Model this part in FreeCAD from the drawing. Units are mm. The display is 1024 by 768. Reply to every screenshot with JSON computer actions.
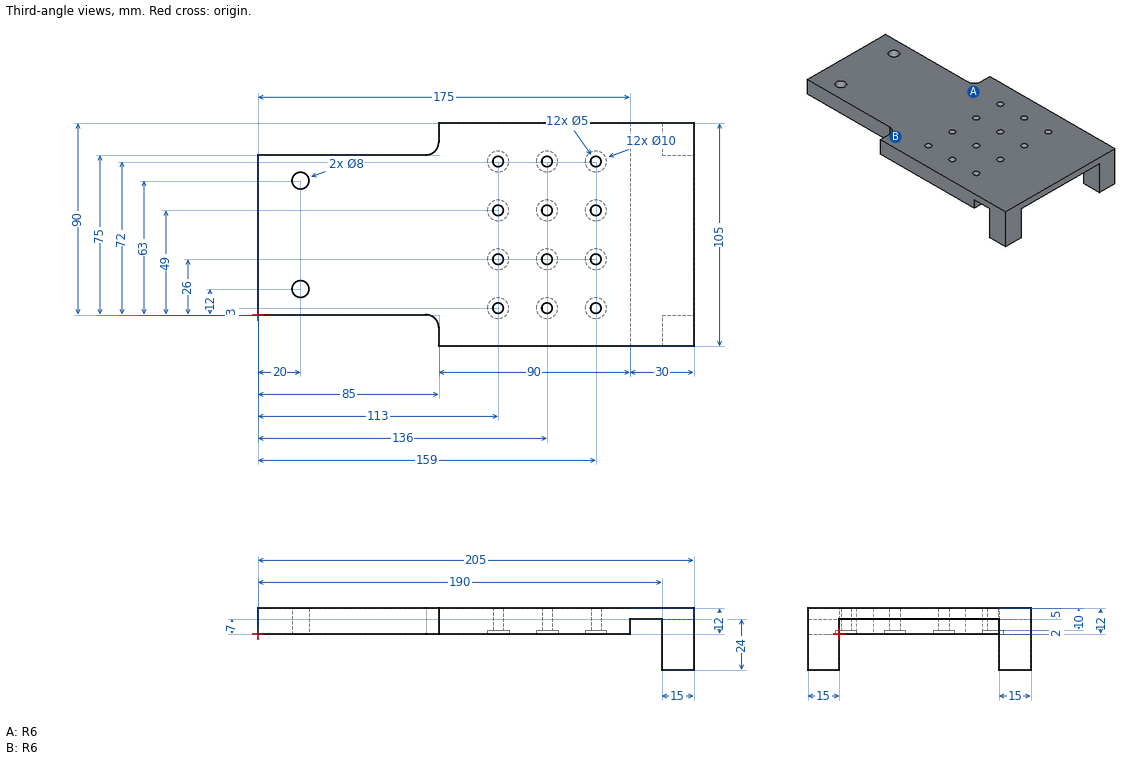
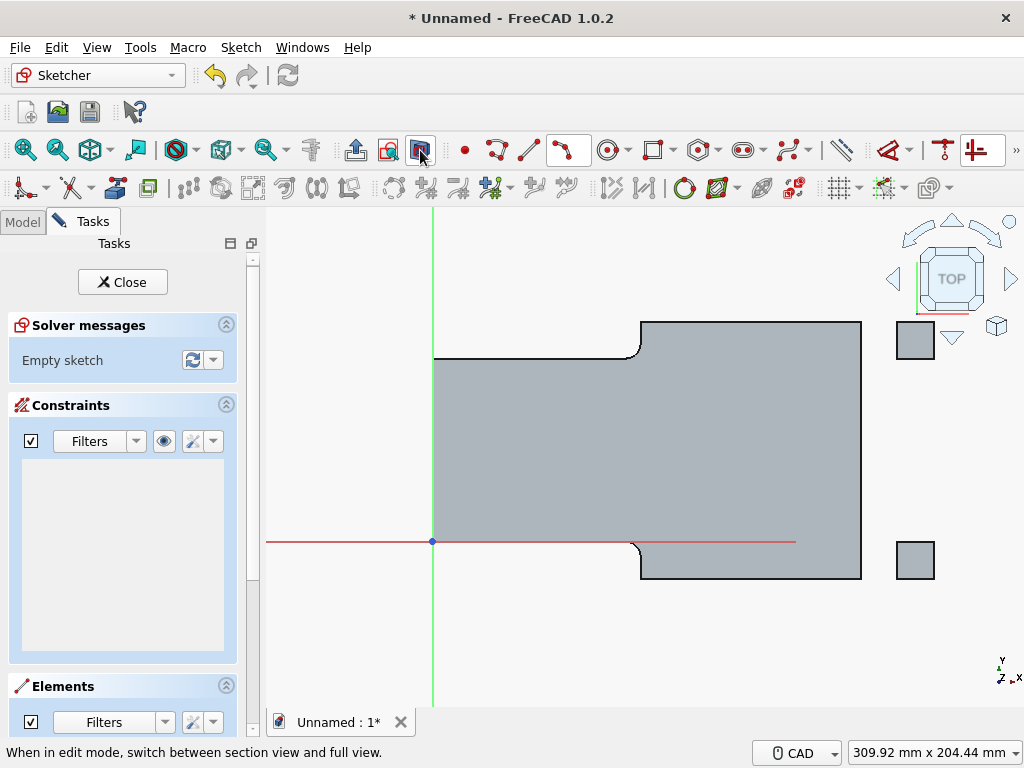
{"action": "left_click", "coordinate": [608, 150]}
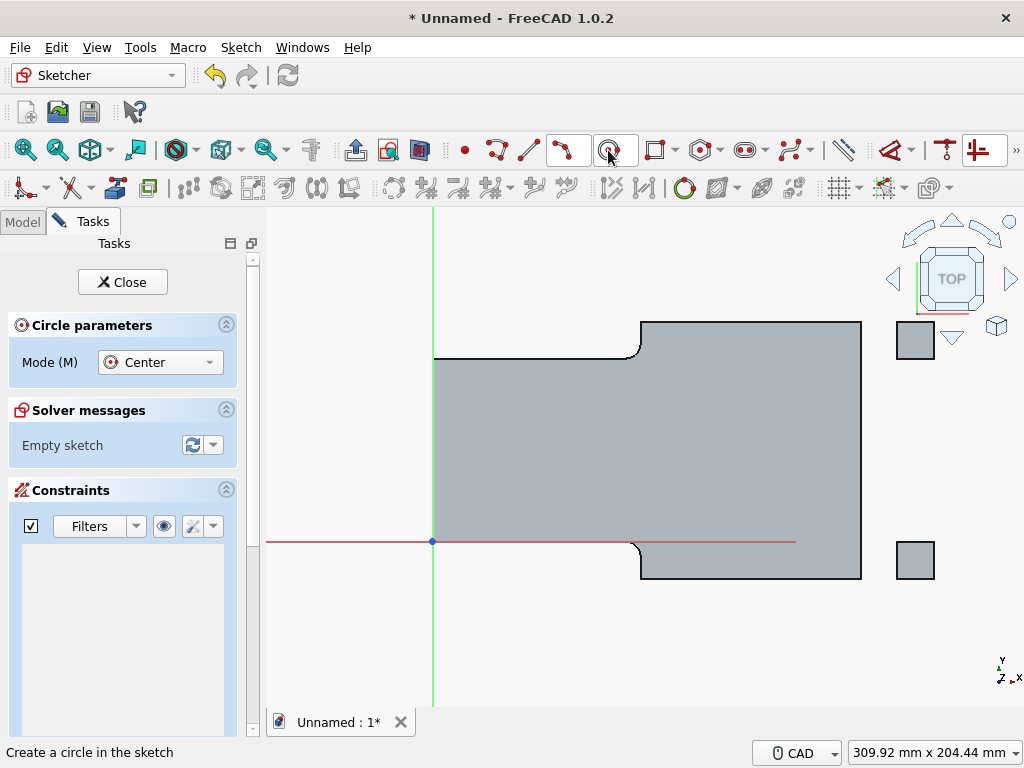
{"action": "scroll", "coordinate": [822, 366], "scroll_direction": "up", "scroll_amount": 4}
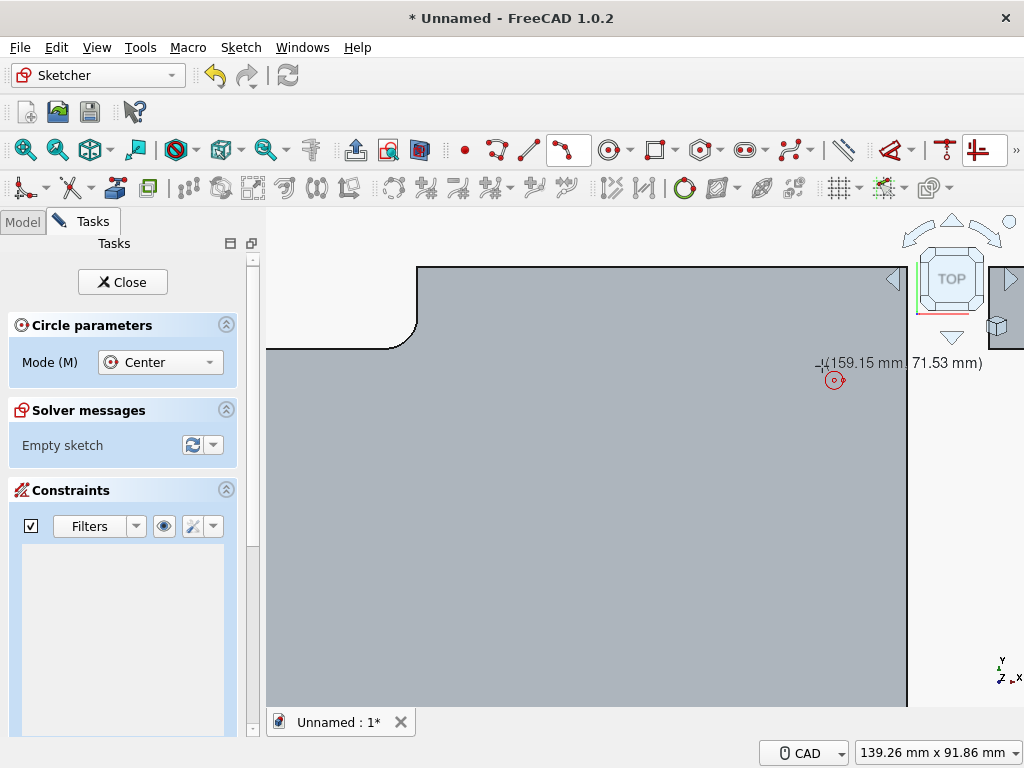
{"action": "left_click", "coordinate": [820, 365]}
{"action": "mouse_move", "coordinate": [840, 346]}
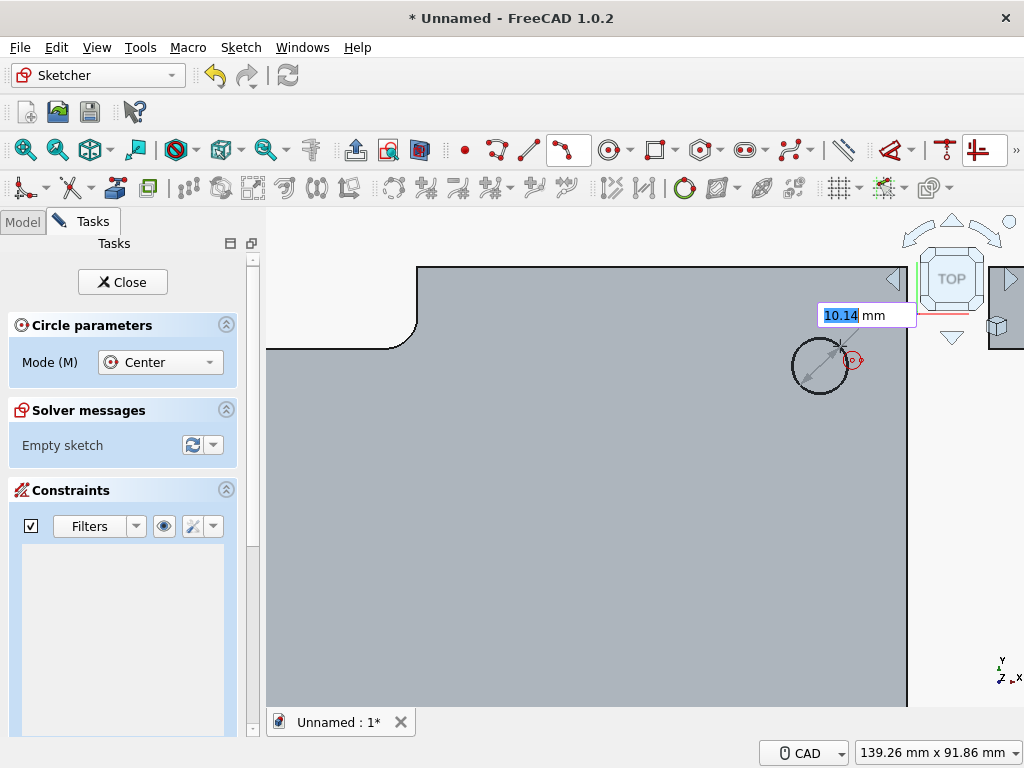
{"action": "type", "text": "10"}
{"action": "key", "text": "Return"}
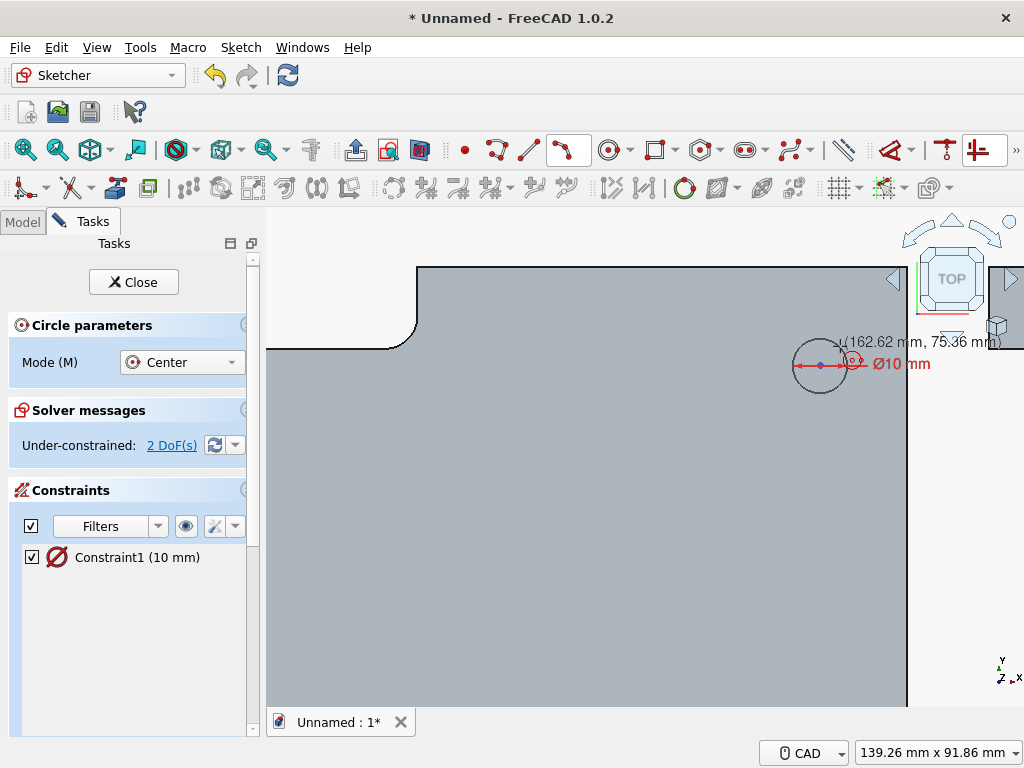
{"action": "left_click", "coordinate": [695, 365]}
{"action": "mouse_move", "coordinate": [714, 346]}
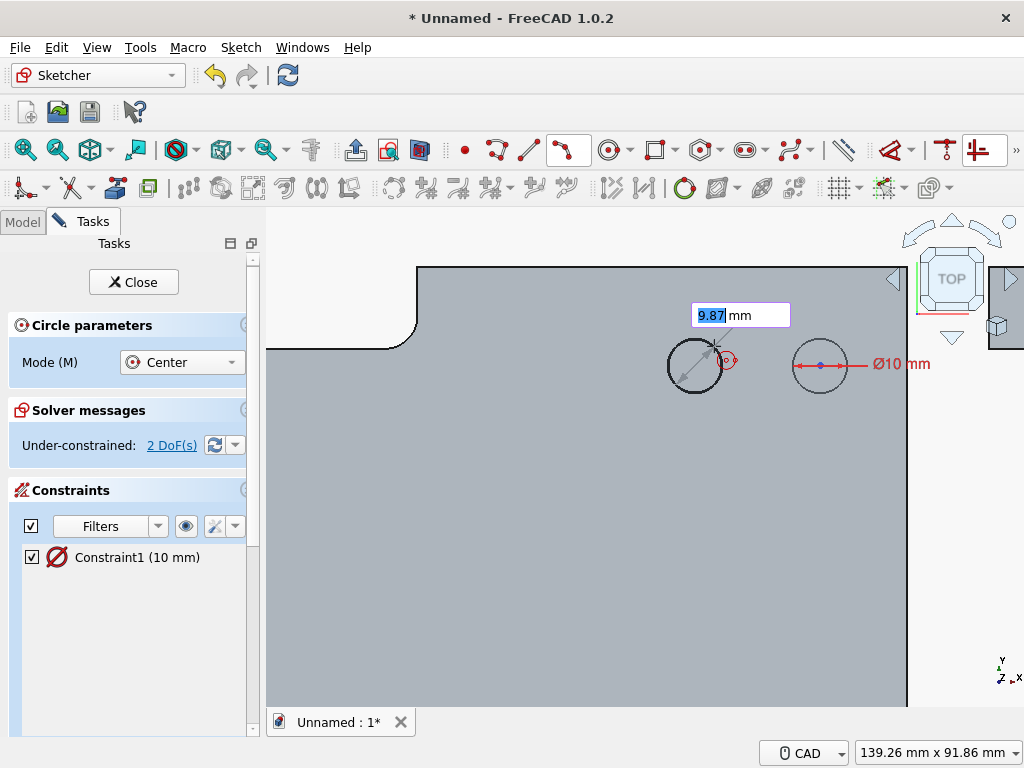
{"action": "type", "text": "10"}
{"action": "key", "text": "Return"}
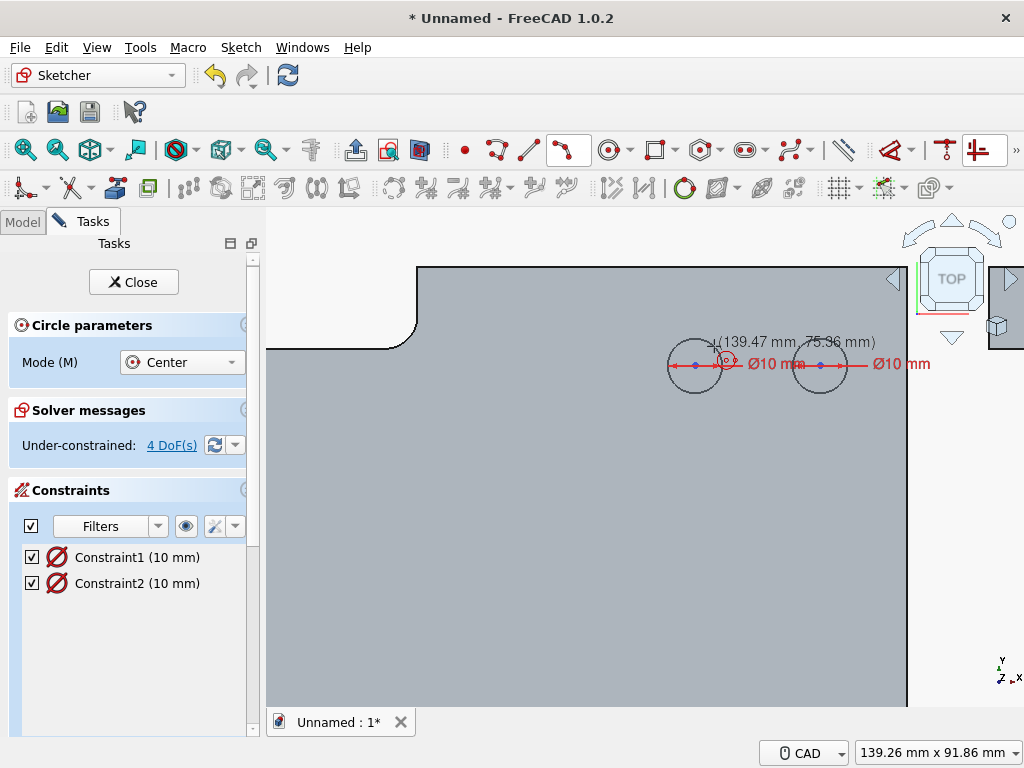
{"action": "left_click", "coordinate": [570, 365]}
{"action": "mouse_move", "coordinate": [589, 346]}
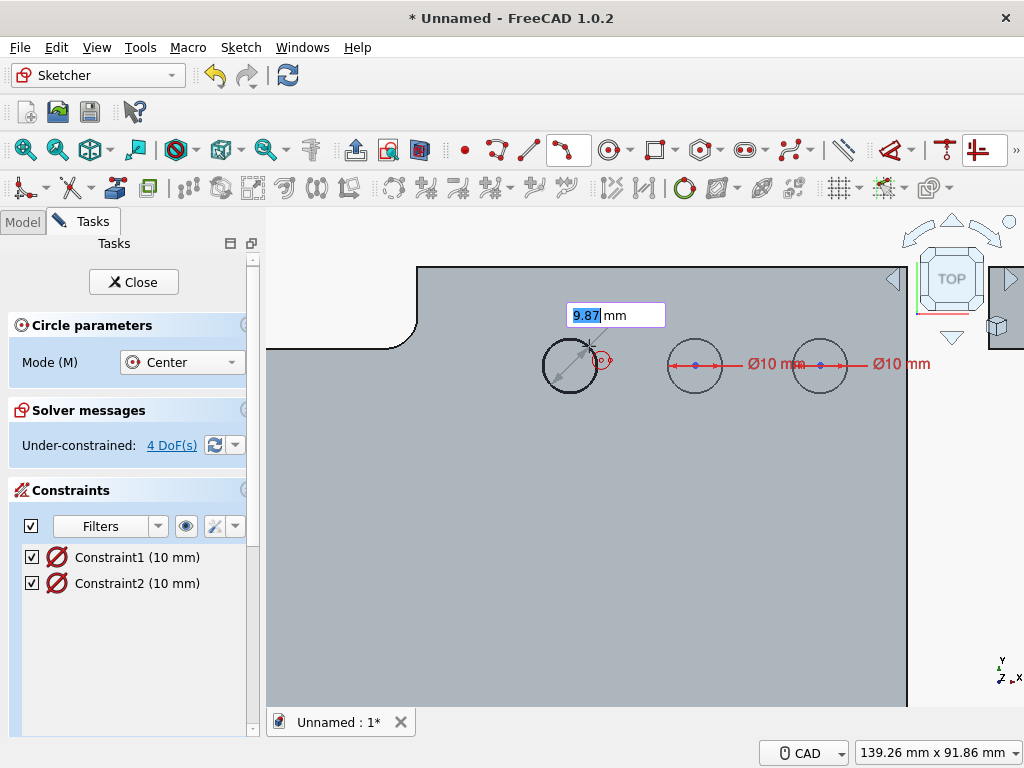
{"action": "type", "text": "10"}
{"action": "key", "text": "Return"}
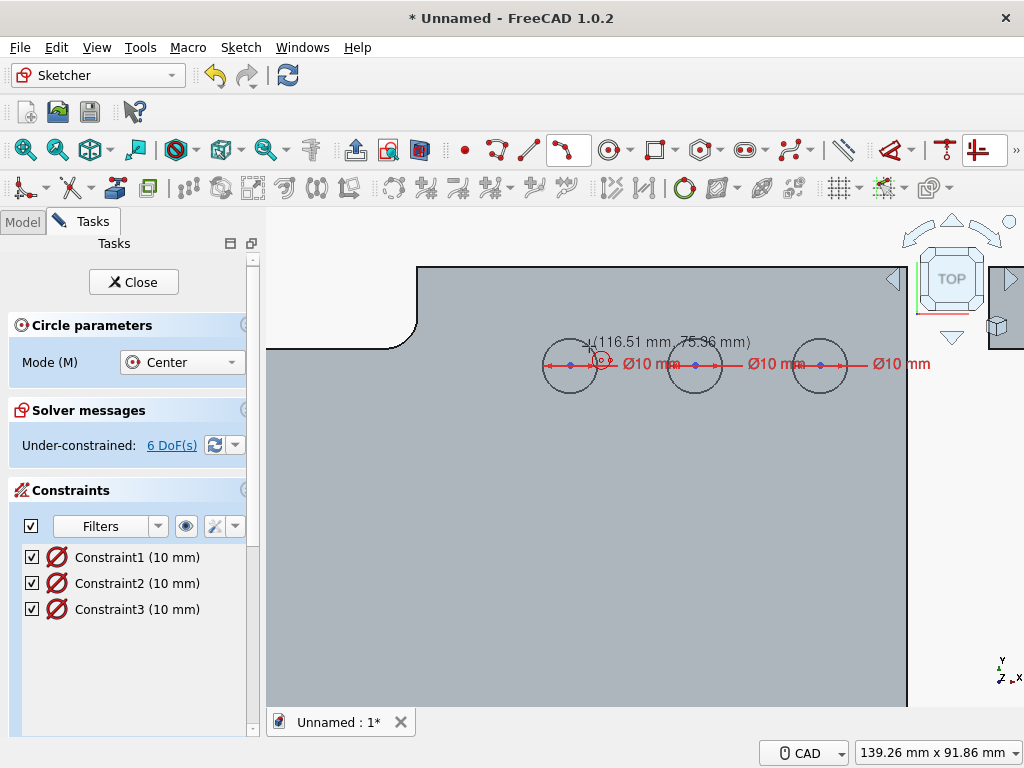
{"action": "left_click", "coordinate": [570, 490]}
{"action": "mouse_move", "coordinate": [589, 471]}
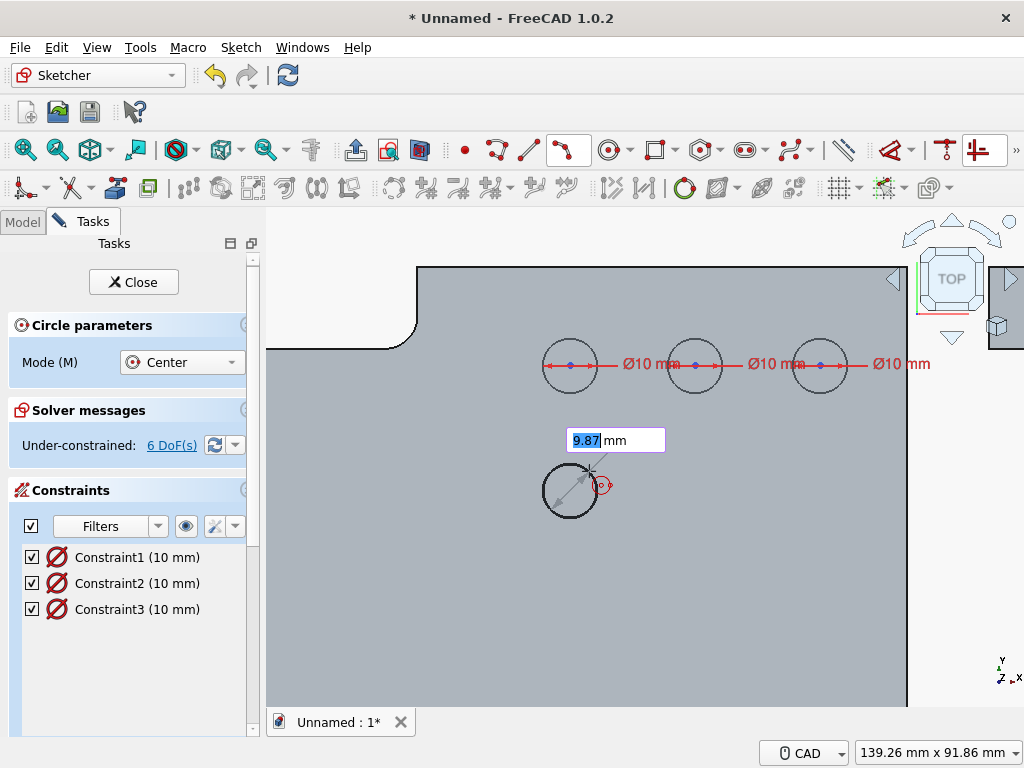
{"action": "type", "text": "10"}
{"action": "key", "text": "Return"}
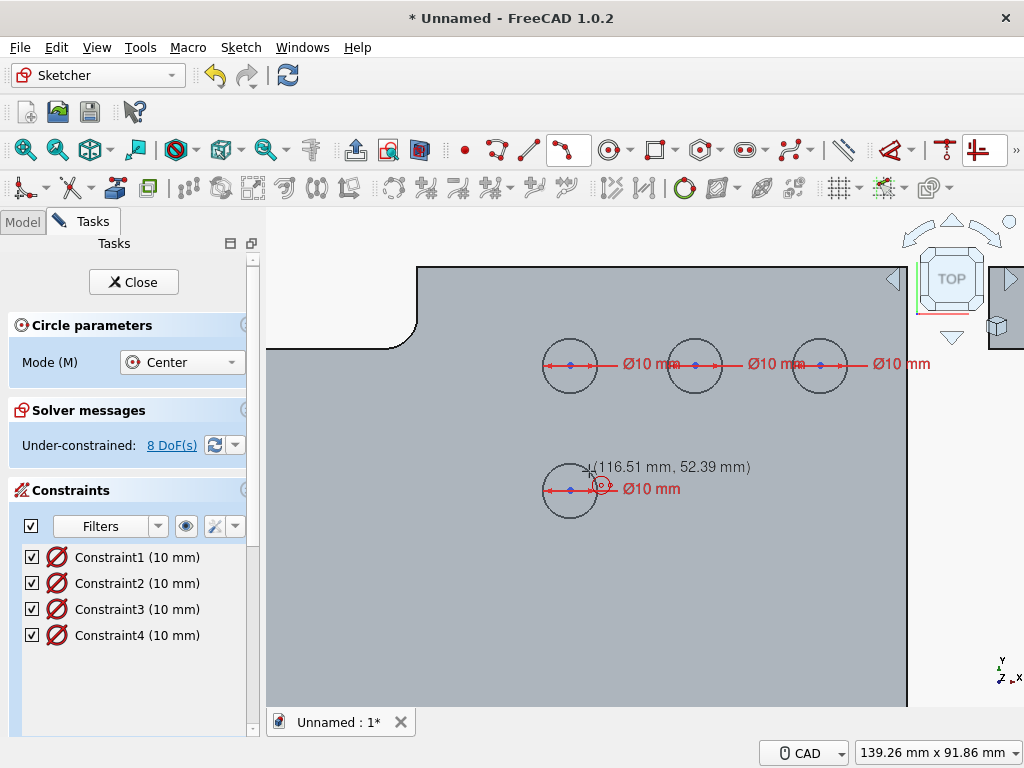
{"action": "left_click", "coordinate": [695, 490]}
{"action": "mouse_move", "coordinate": [714, 471]}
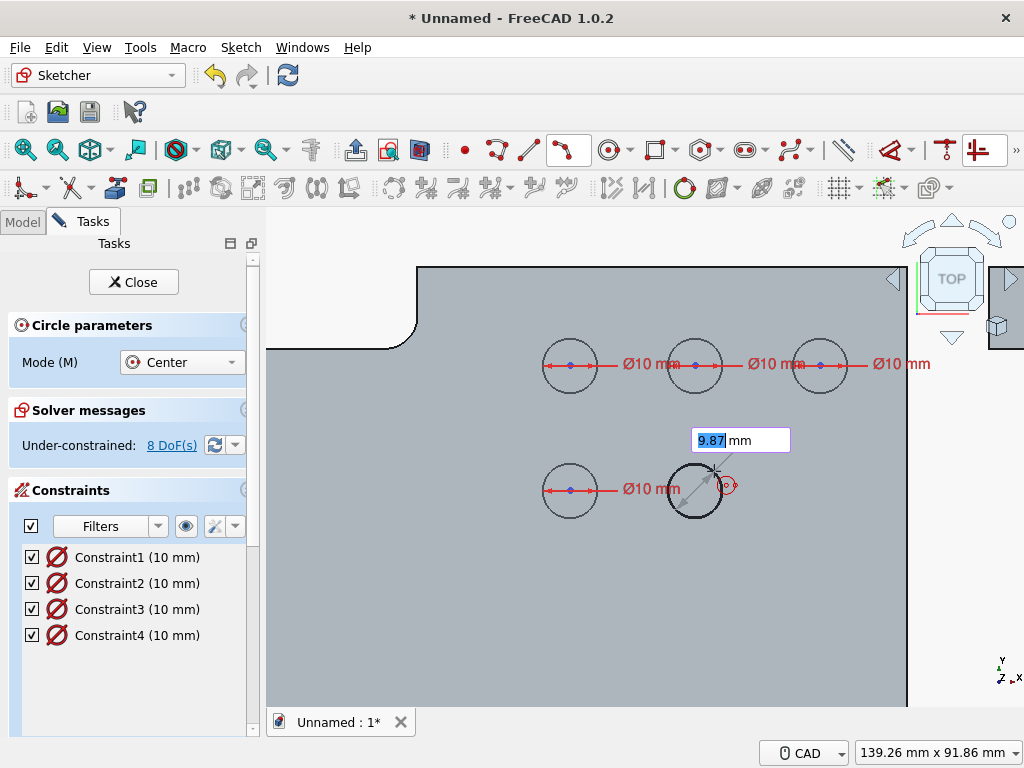
{"action": "type", "text": "10"}
{"action": "key", "text": "Return"}